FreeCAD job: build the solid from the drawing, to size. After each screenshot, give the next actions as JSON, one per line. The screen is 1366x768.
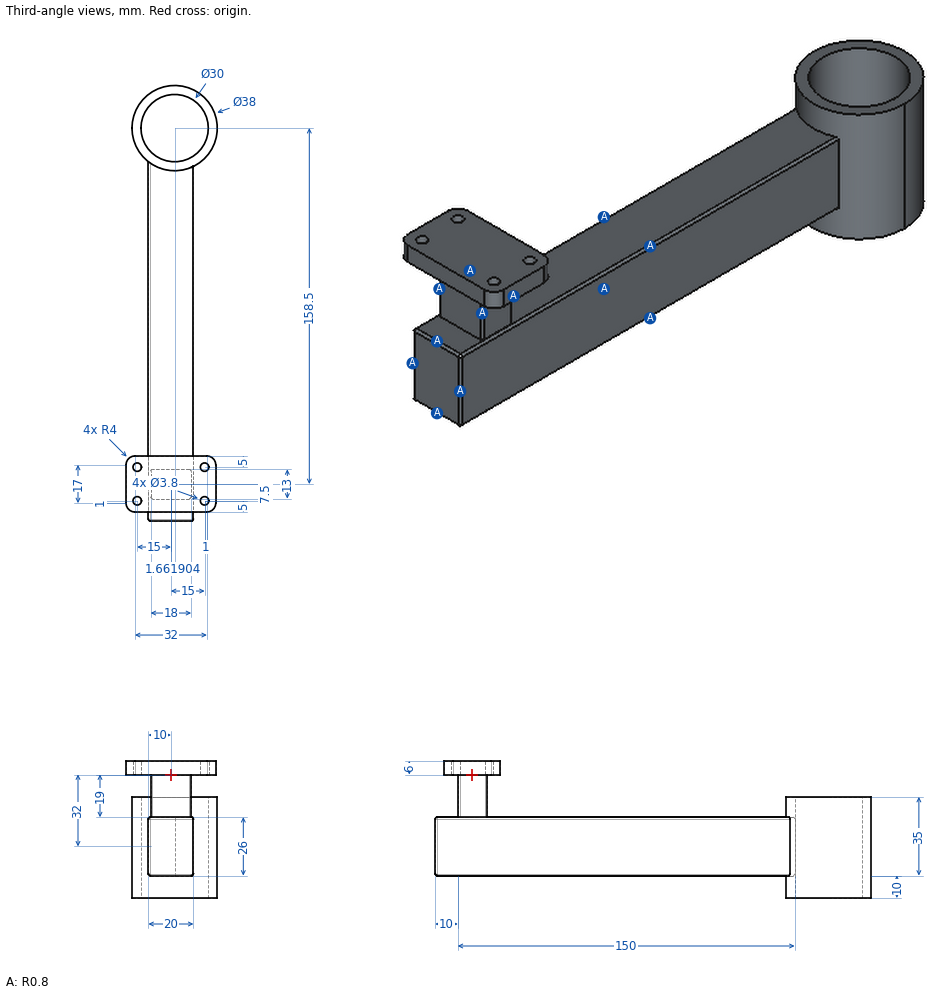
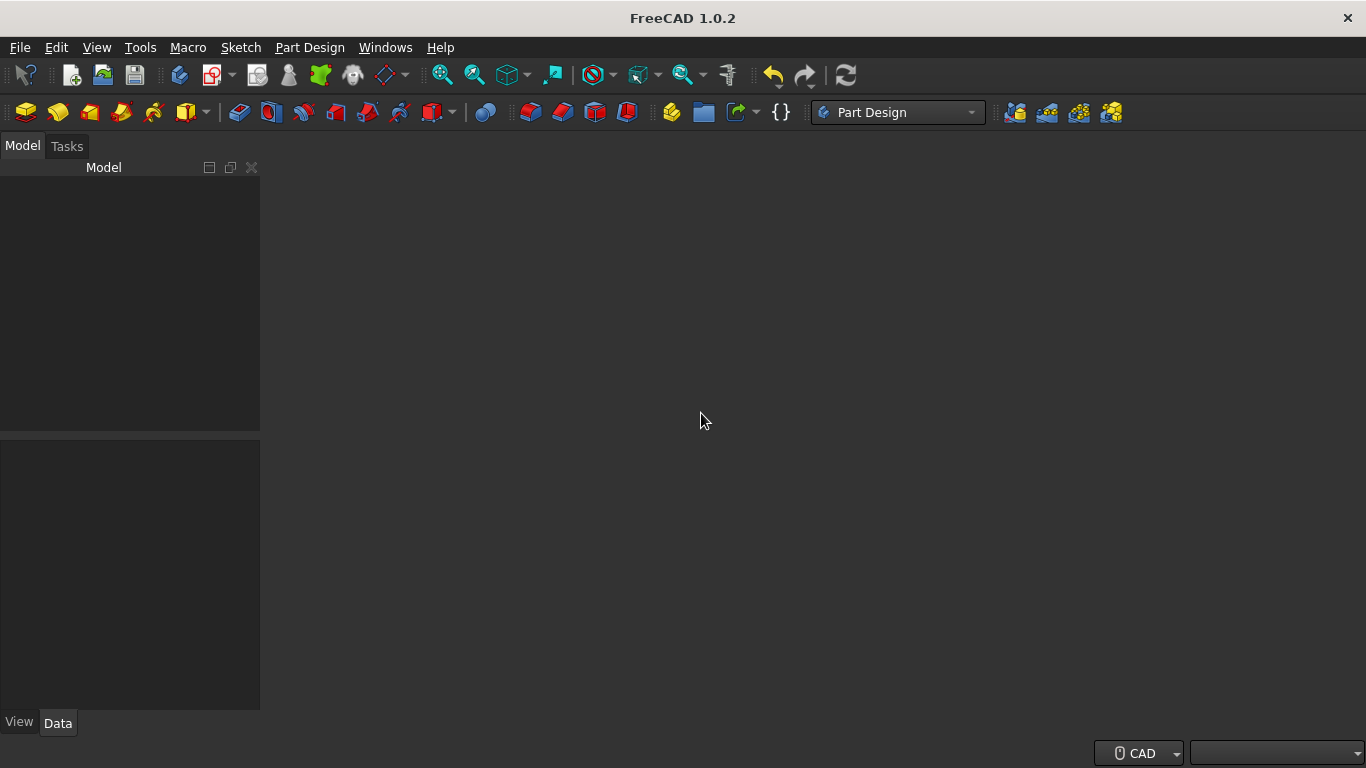
{"action": "key", "text": "ctrl+n"}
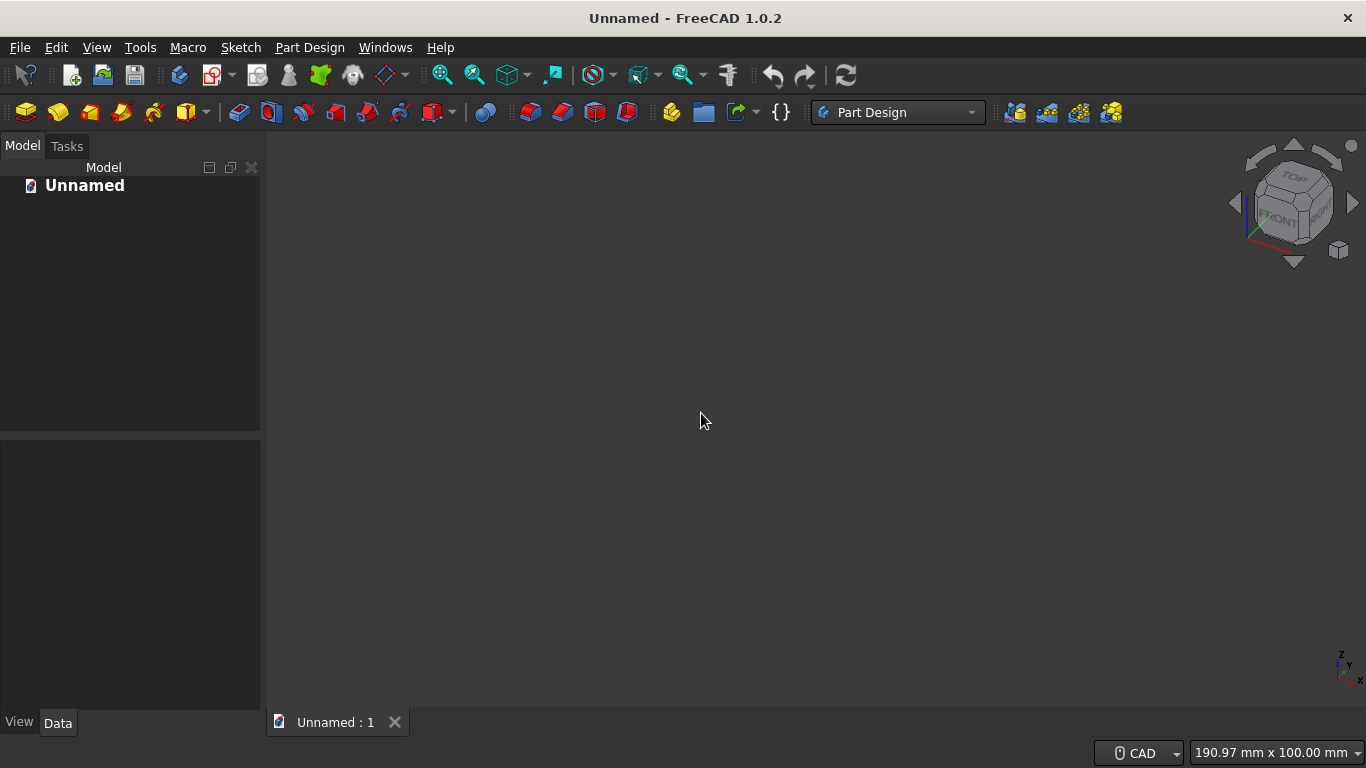
{"action": "left_click", "coordinate": [212, 76]}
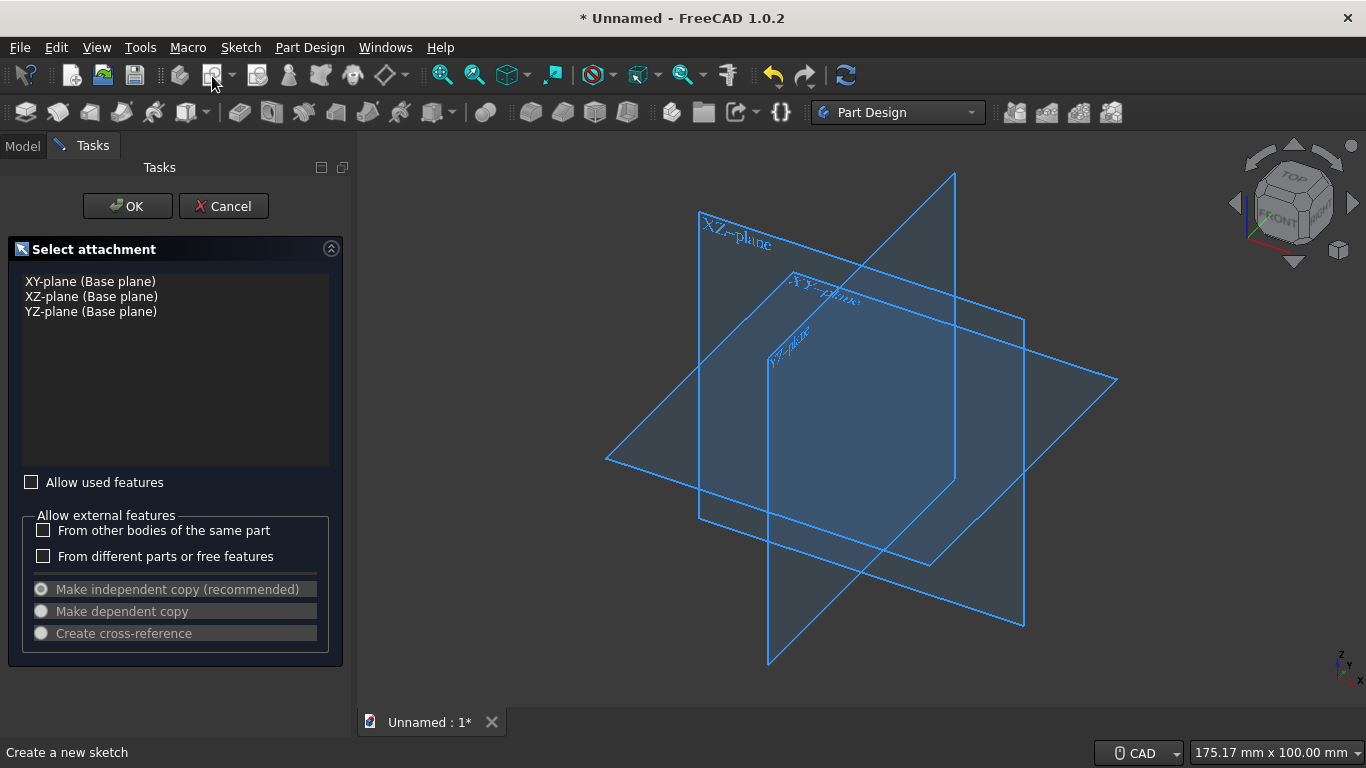
{"action": "left_click", "coordinate": [82, 282]}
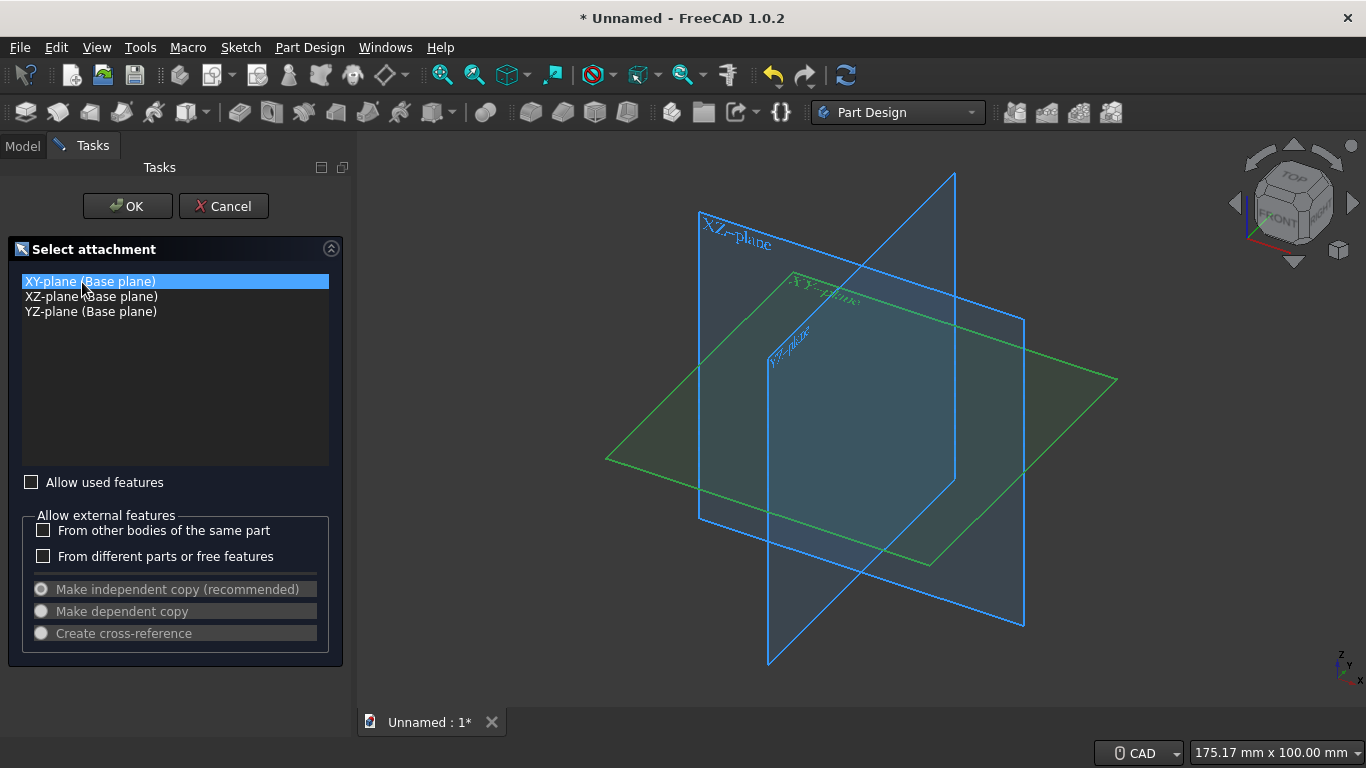
{"action": "left_click", "coordinate": [128, 206]}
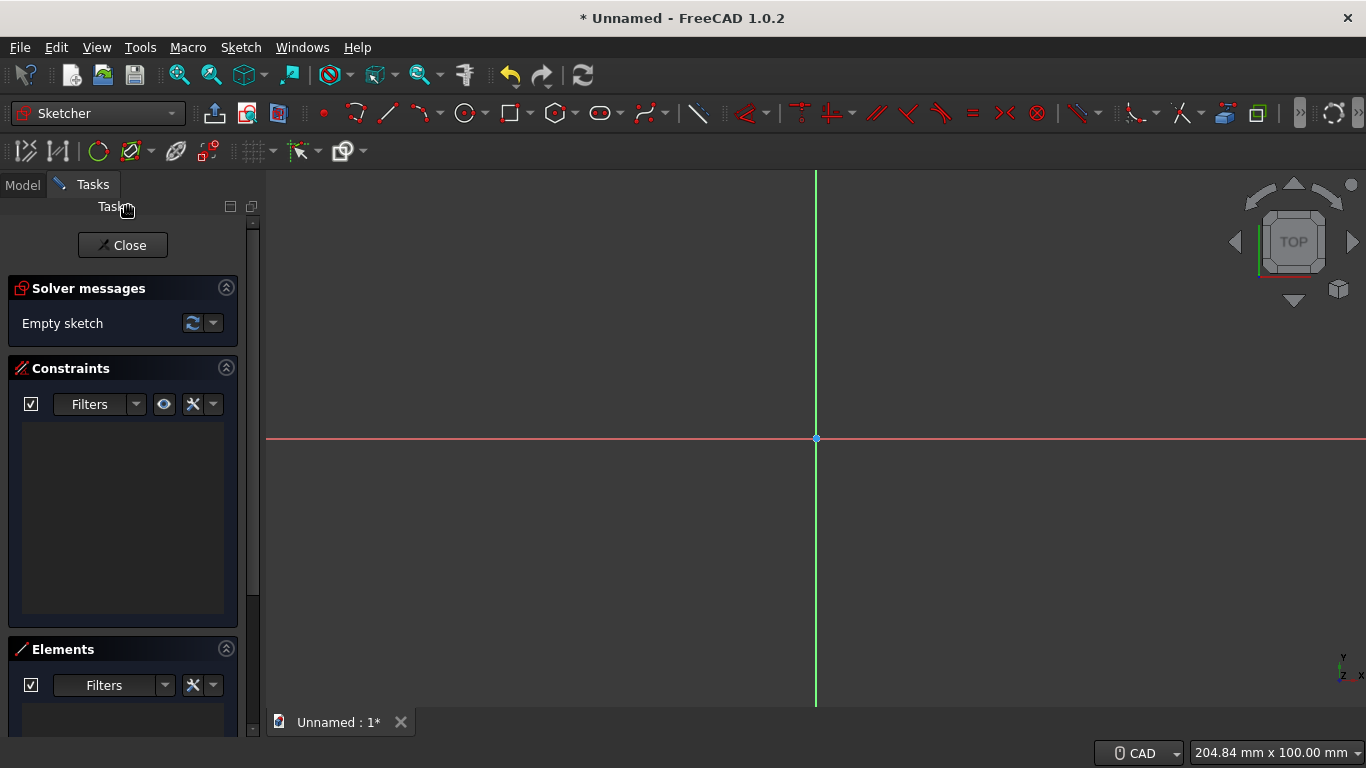
{"action": "scroll", "coordinate": [856, 439], "scroll_direction": "up", "scroll_amount": 5}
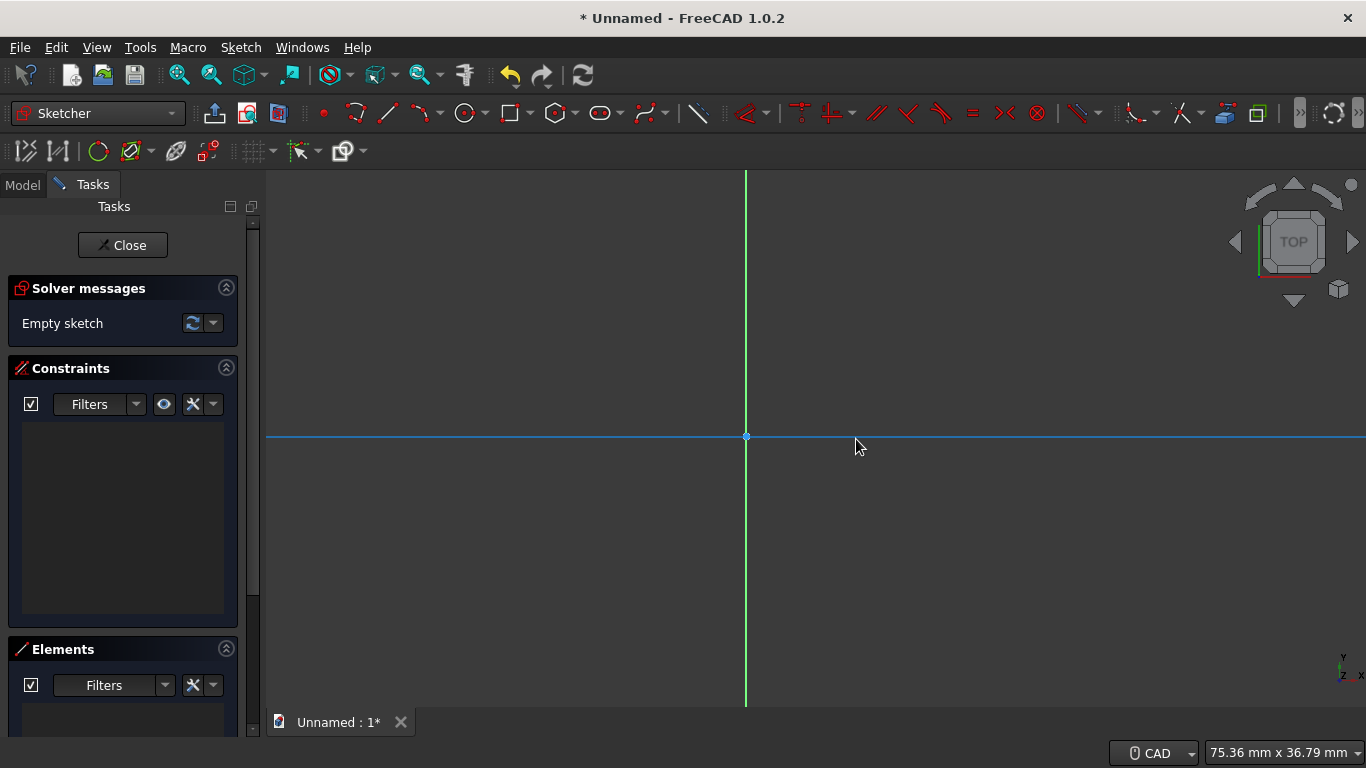
{"action": "left_click", "coordinate": [388, 114]}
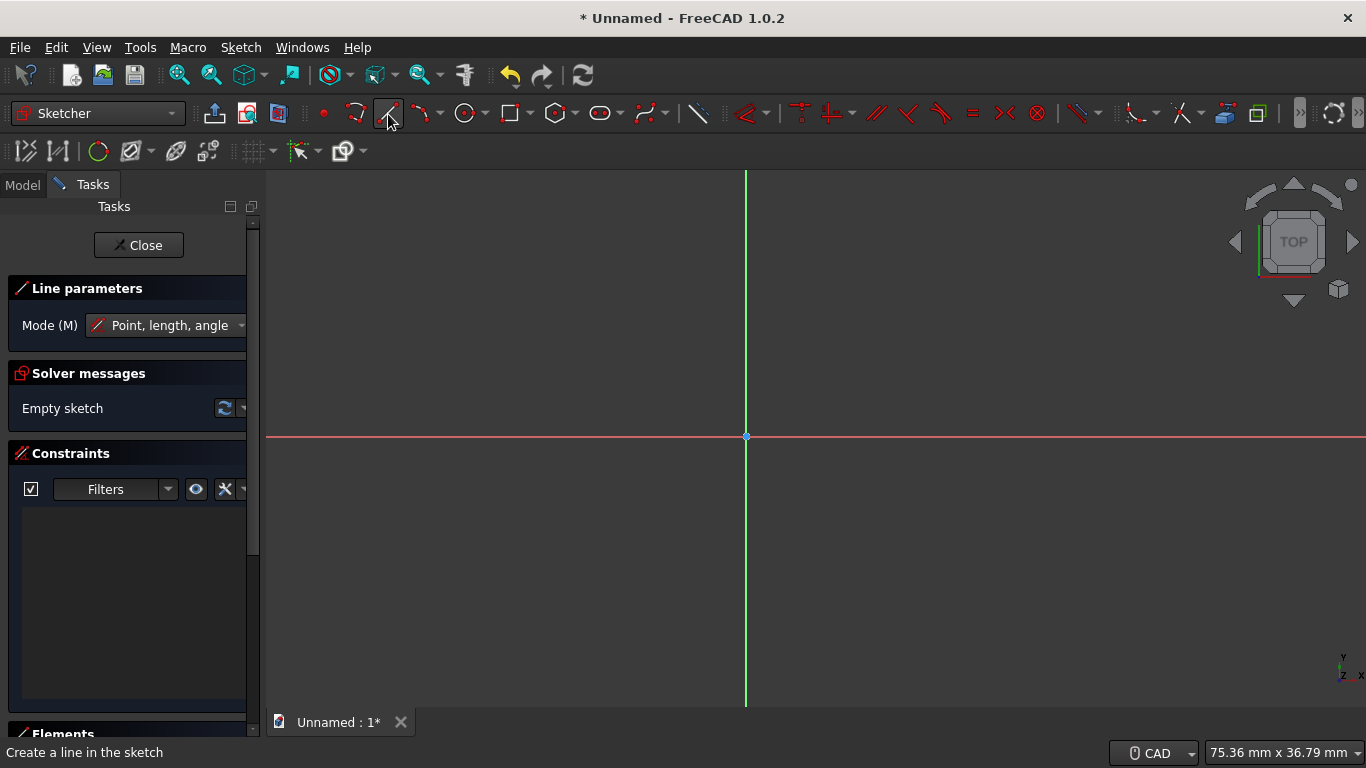
{"action": "left_click", "coordinate": [980, 254]}
{"action": "left_click", "coordinate": [513, 254]}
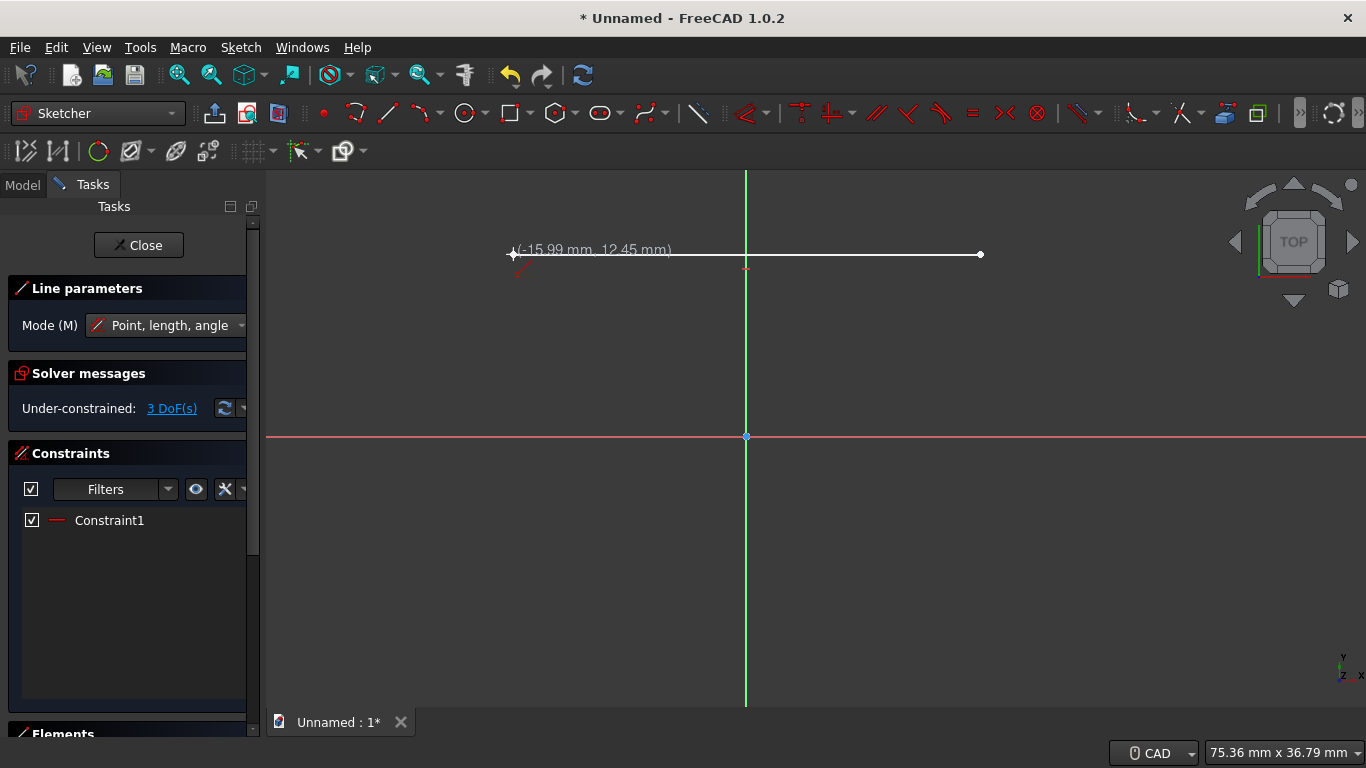
{"action": "left_click", "coordinate": [454, 313]}
{"action": "left_click", "coordinate": [454, 561]}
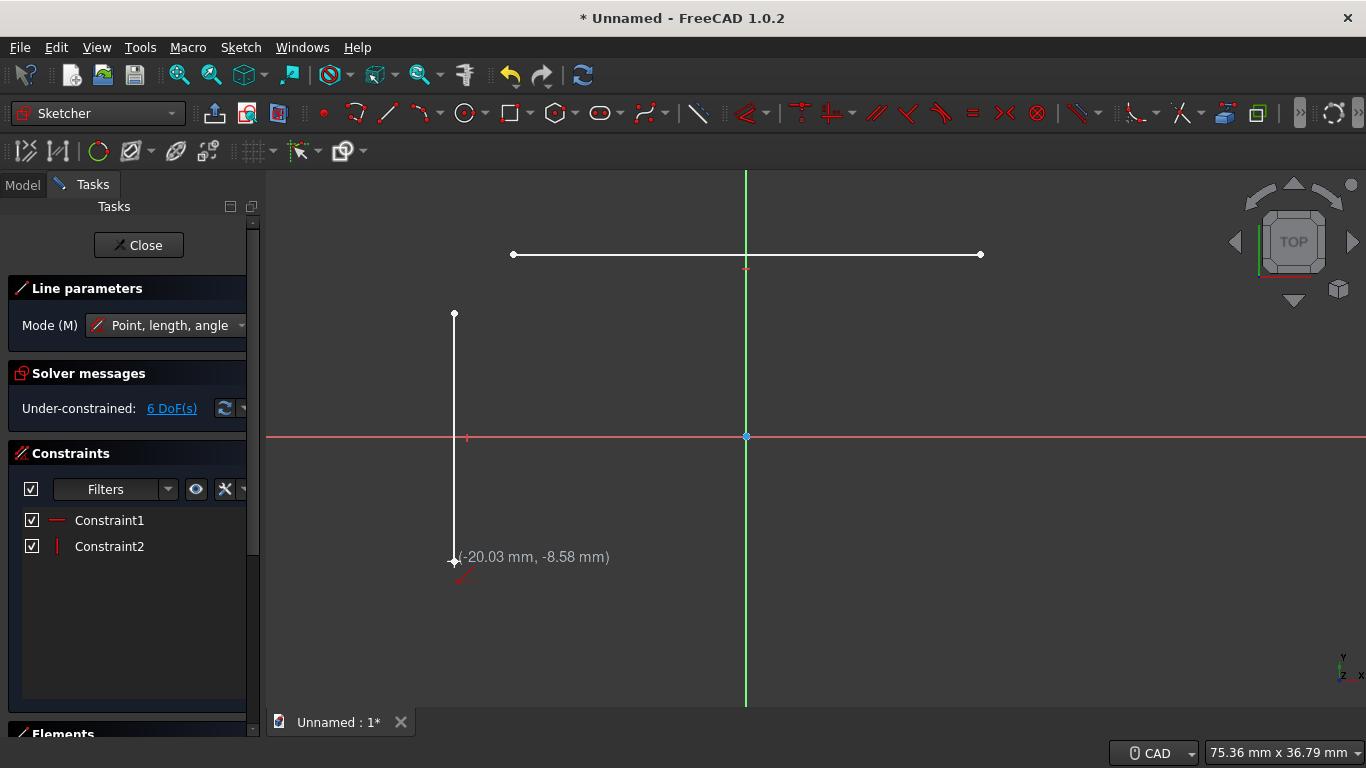
{"action": "left_click", "coordinate": [513, 619]}
{"action": "left_click", "coordinate": [980, 619]}